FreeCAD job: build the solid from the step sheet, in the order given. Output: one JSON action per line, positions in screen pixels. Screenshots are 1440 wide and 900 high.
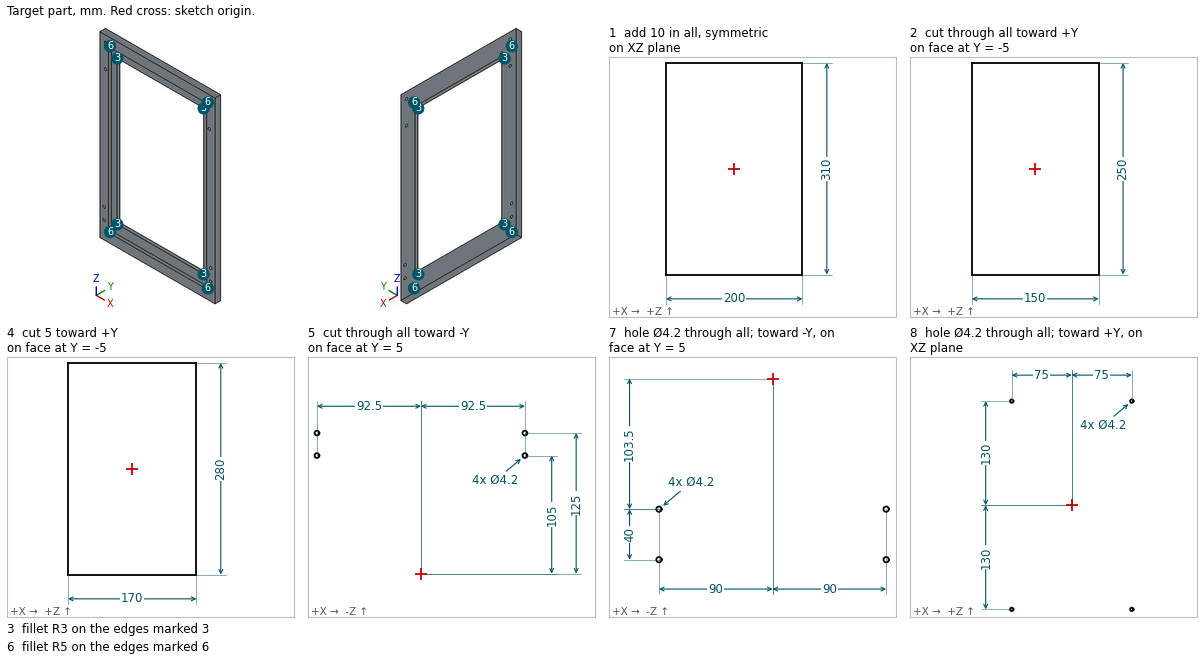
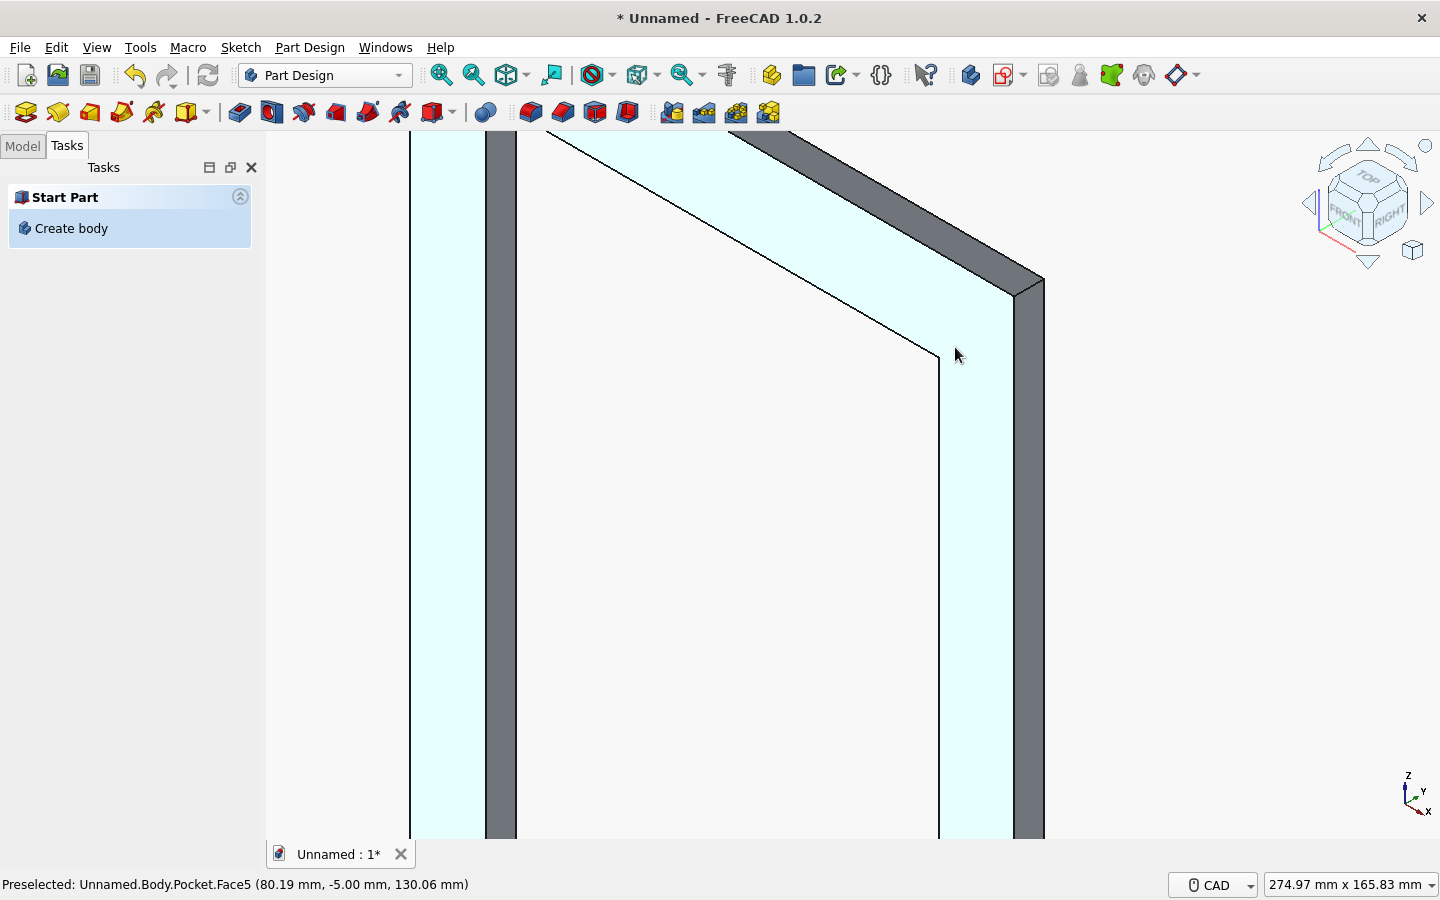
{"action": "key", "text": "v f"}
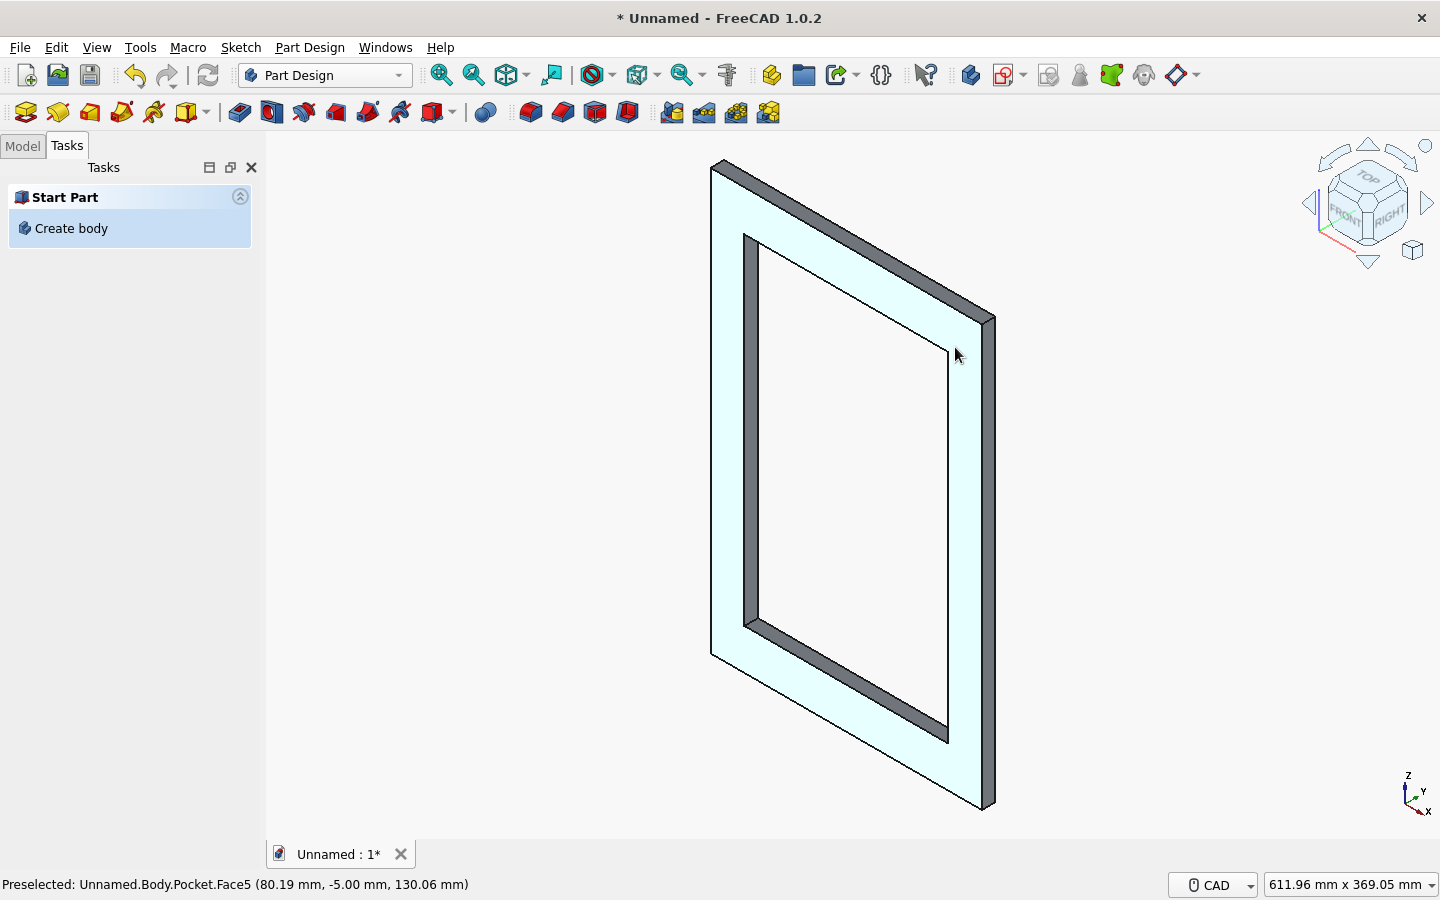
{"action": "key", "text": "2"}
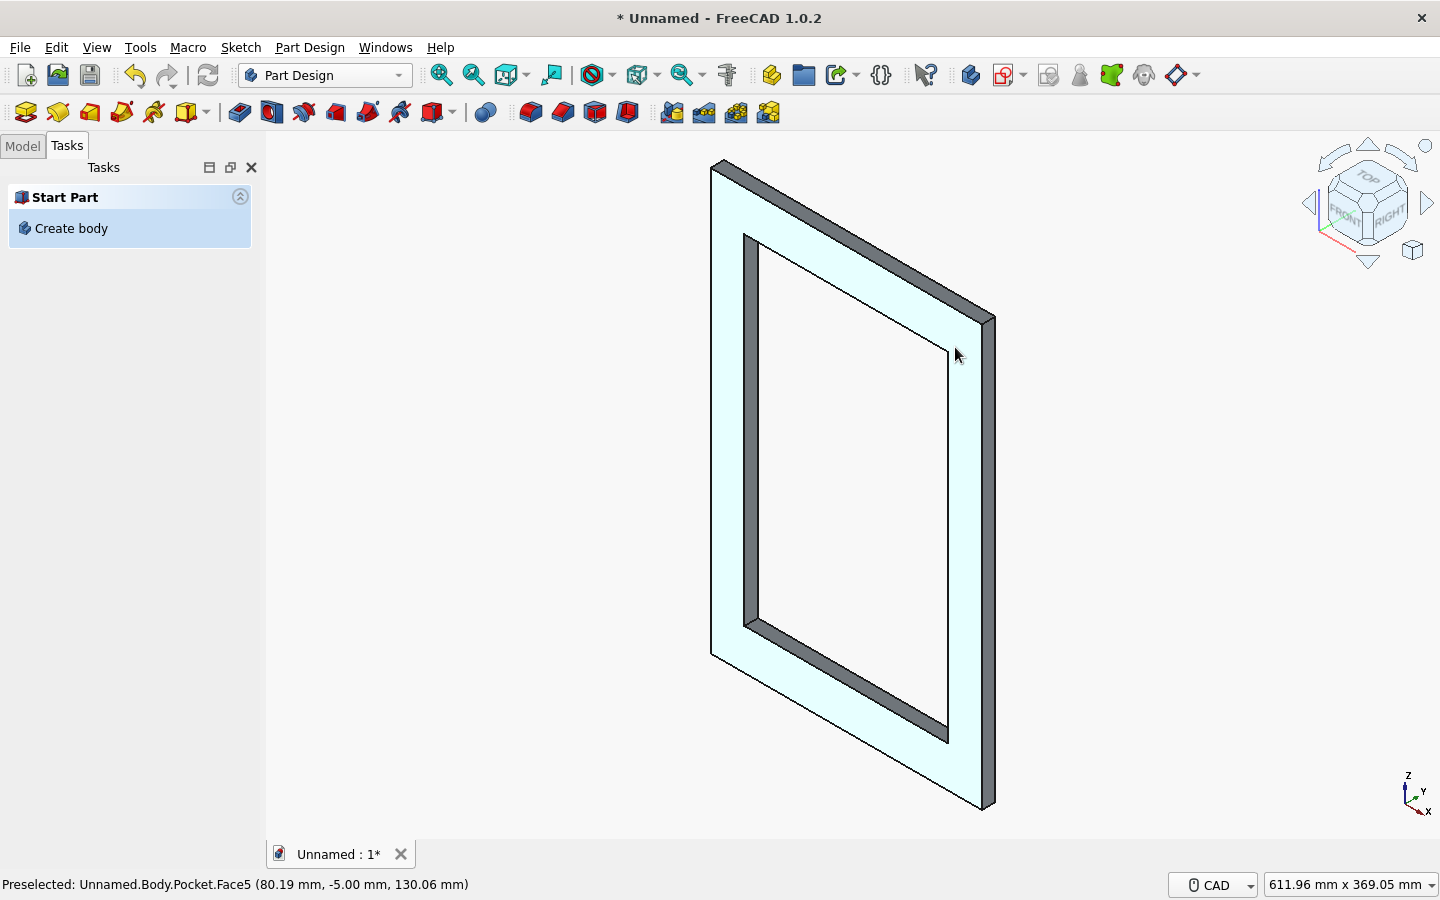
{"action": "key", "text": "v f"}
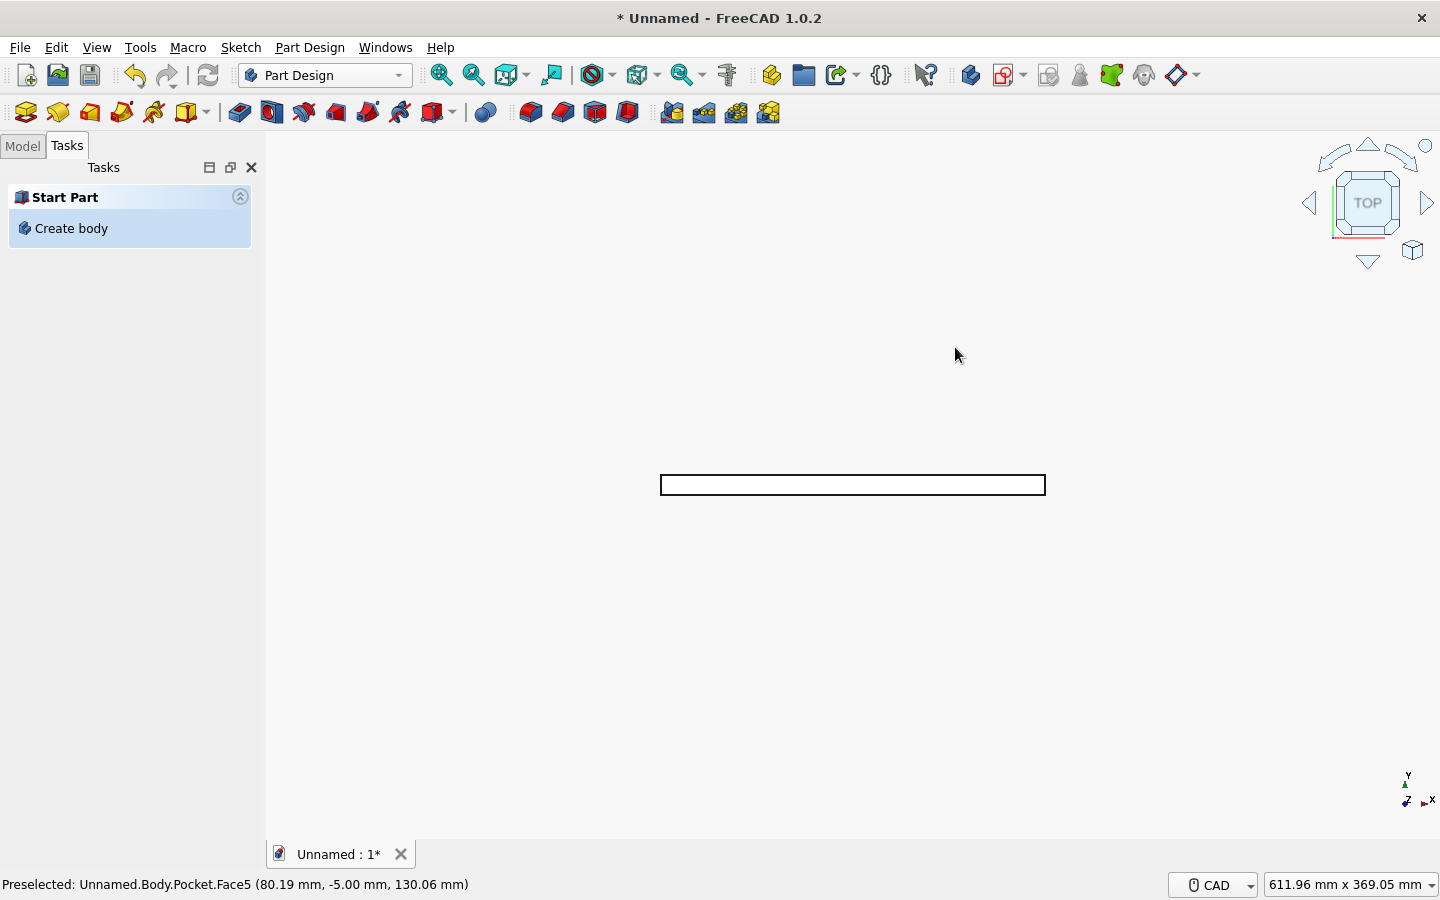
{"action": "scroll", "coordinate": [997, 484], "scroll_direction": "up", "scroll_amount": 4}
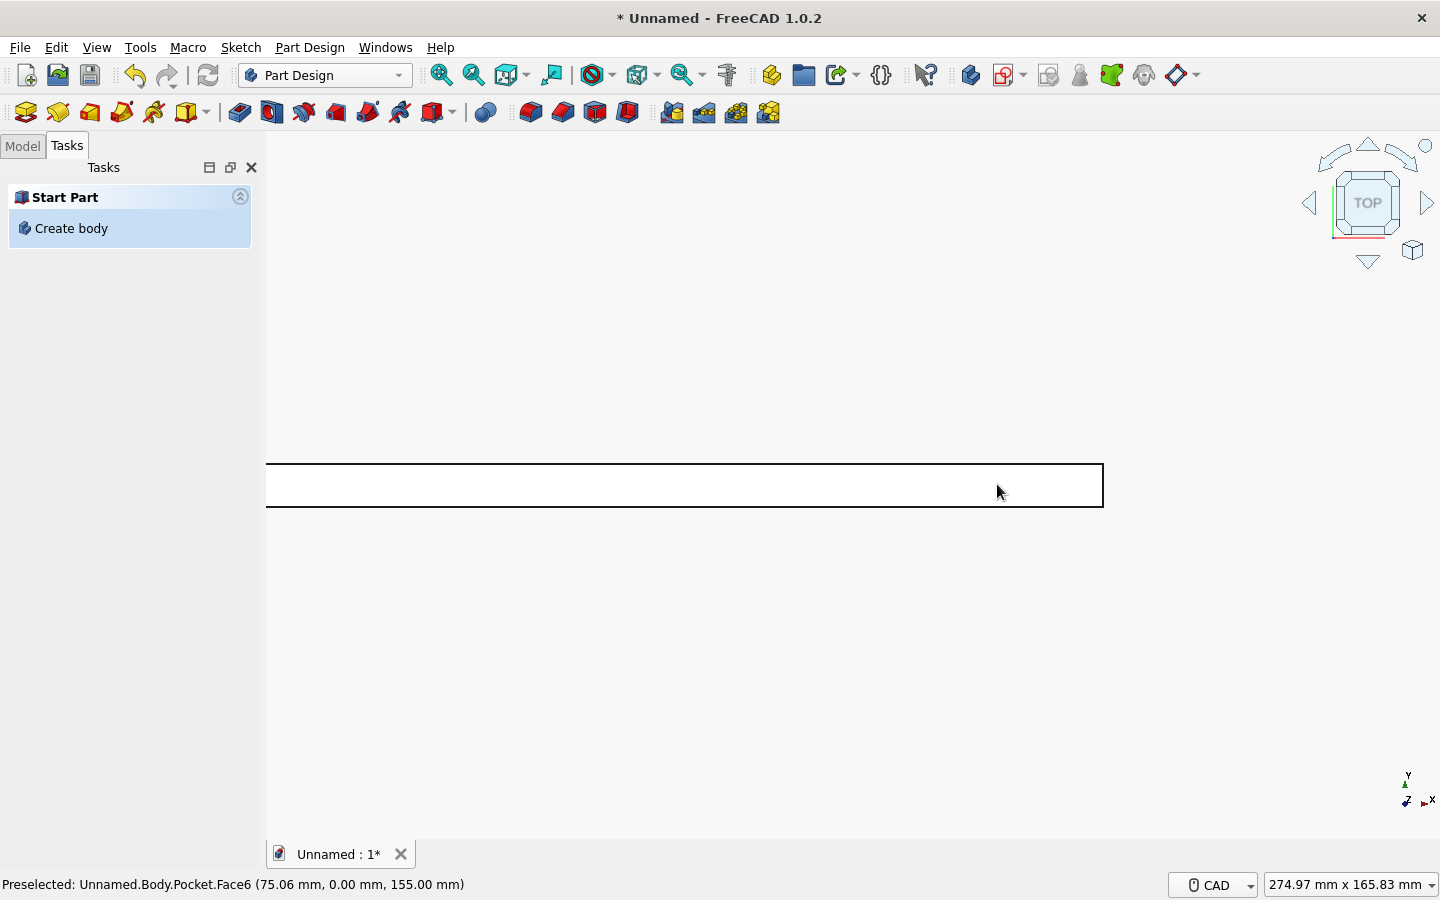
{"action": "key", "text": "v f"}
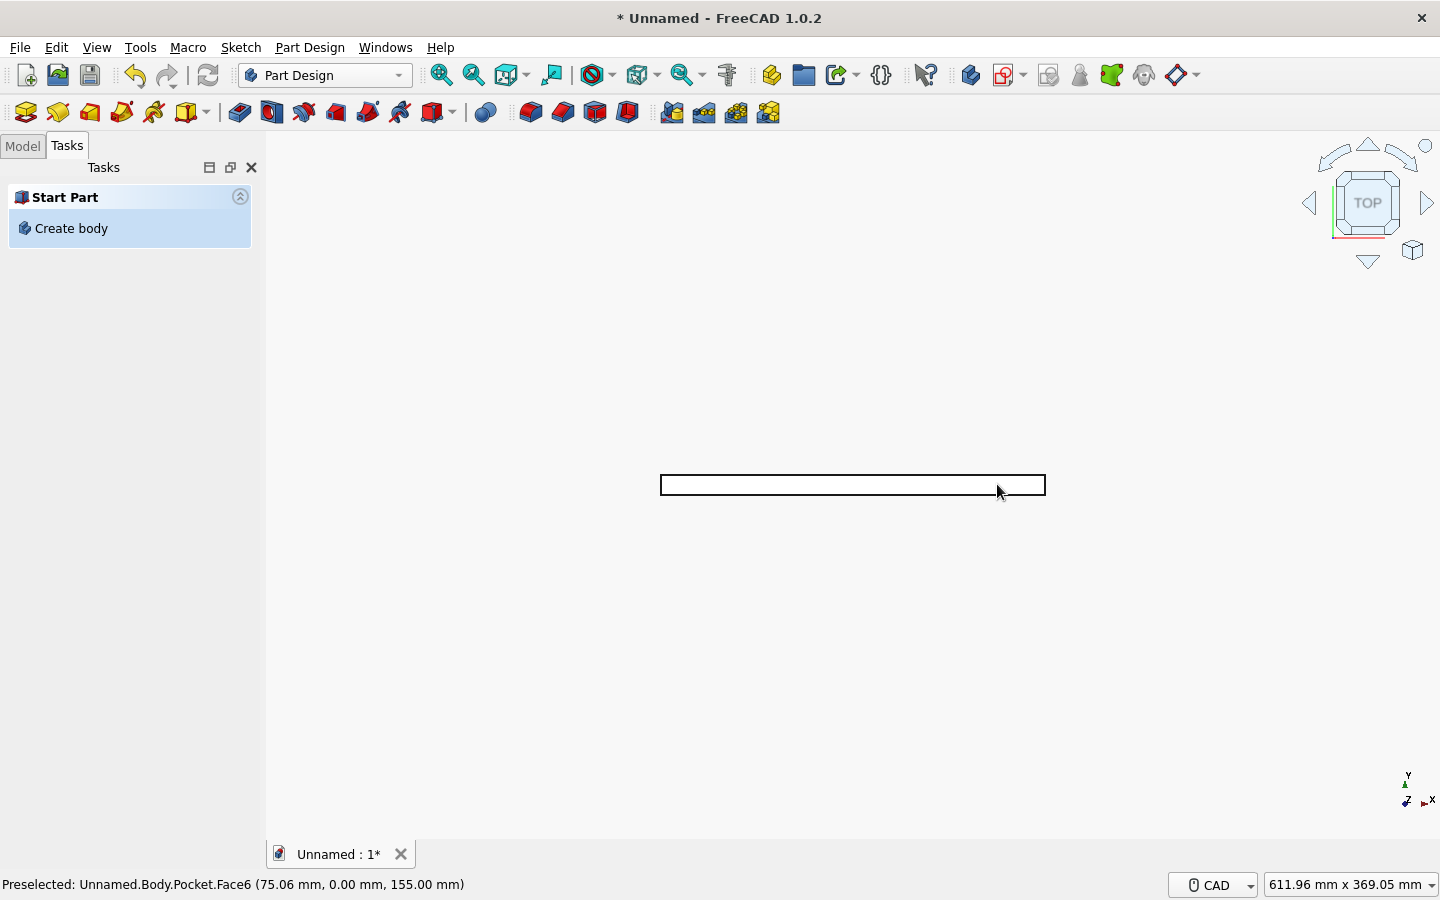
{"action": "key", "text": "1"}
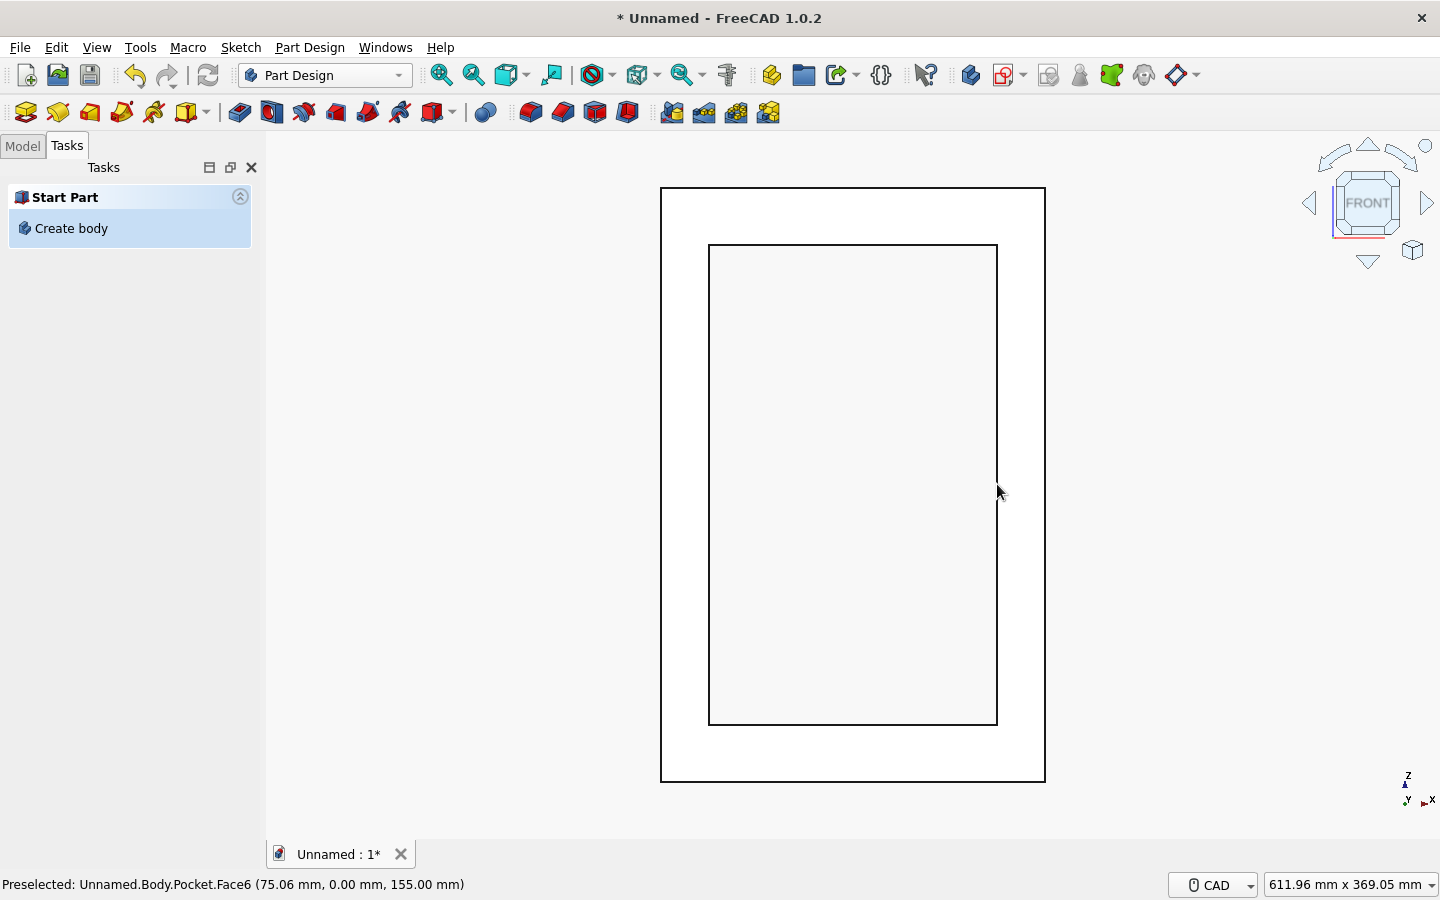
{"action": "scroll", "coordinate": [997, 244], "scroll_direction": "up", "scroll_amount": 4}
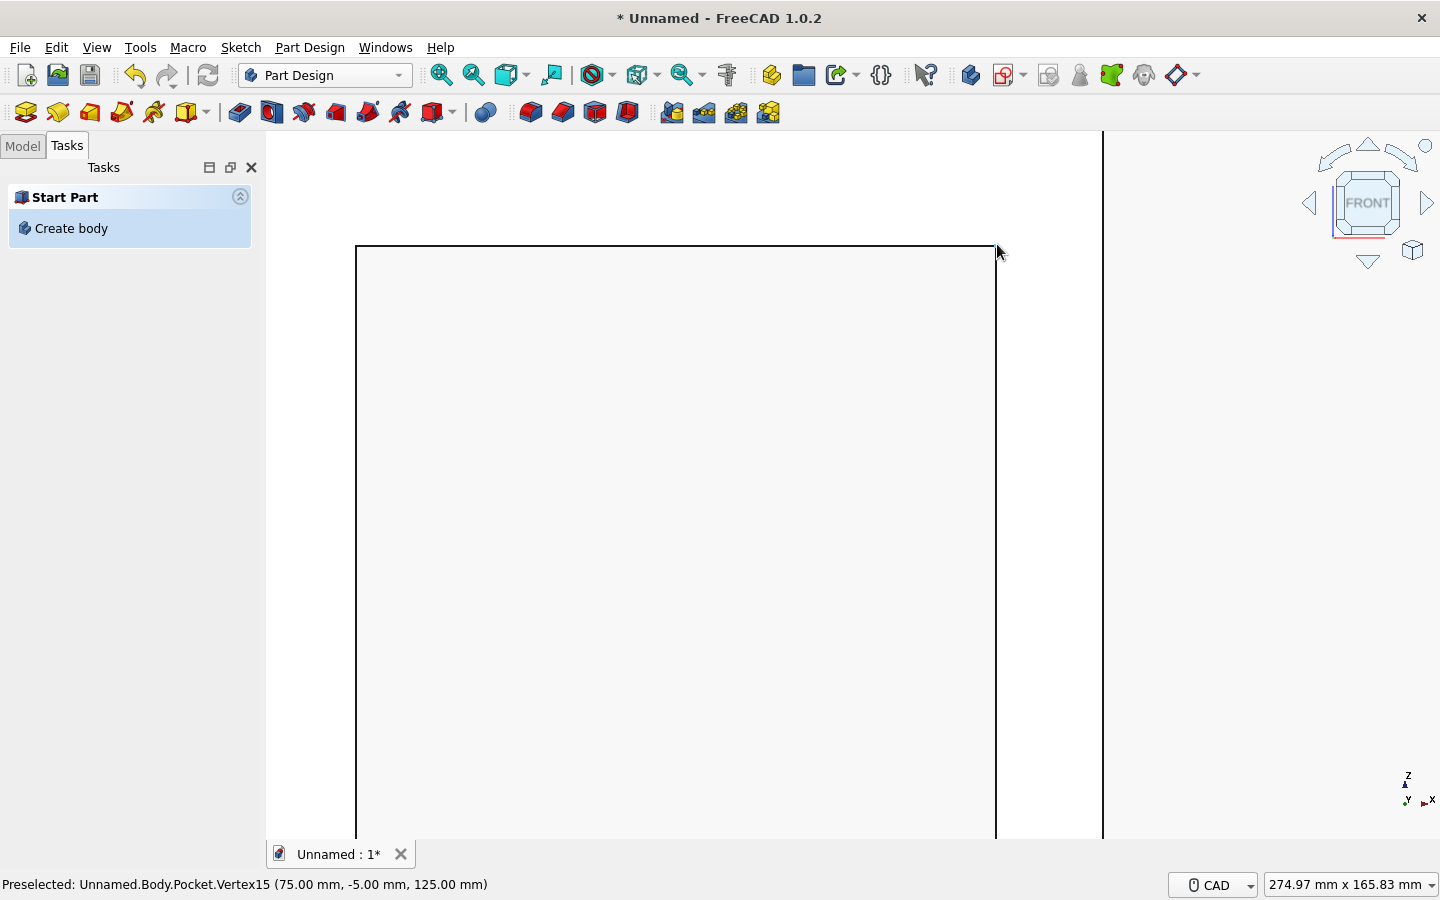
{"action": "key", "text": "v f"}